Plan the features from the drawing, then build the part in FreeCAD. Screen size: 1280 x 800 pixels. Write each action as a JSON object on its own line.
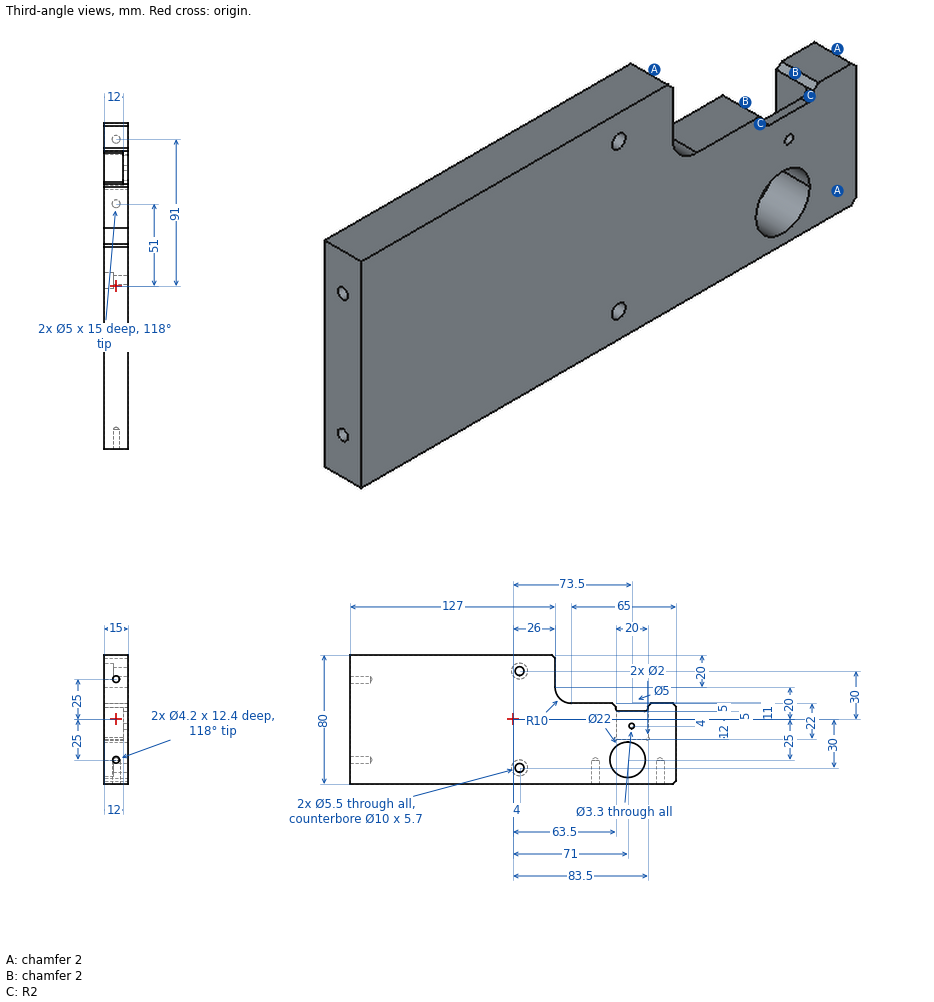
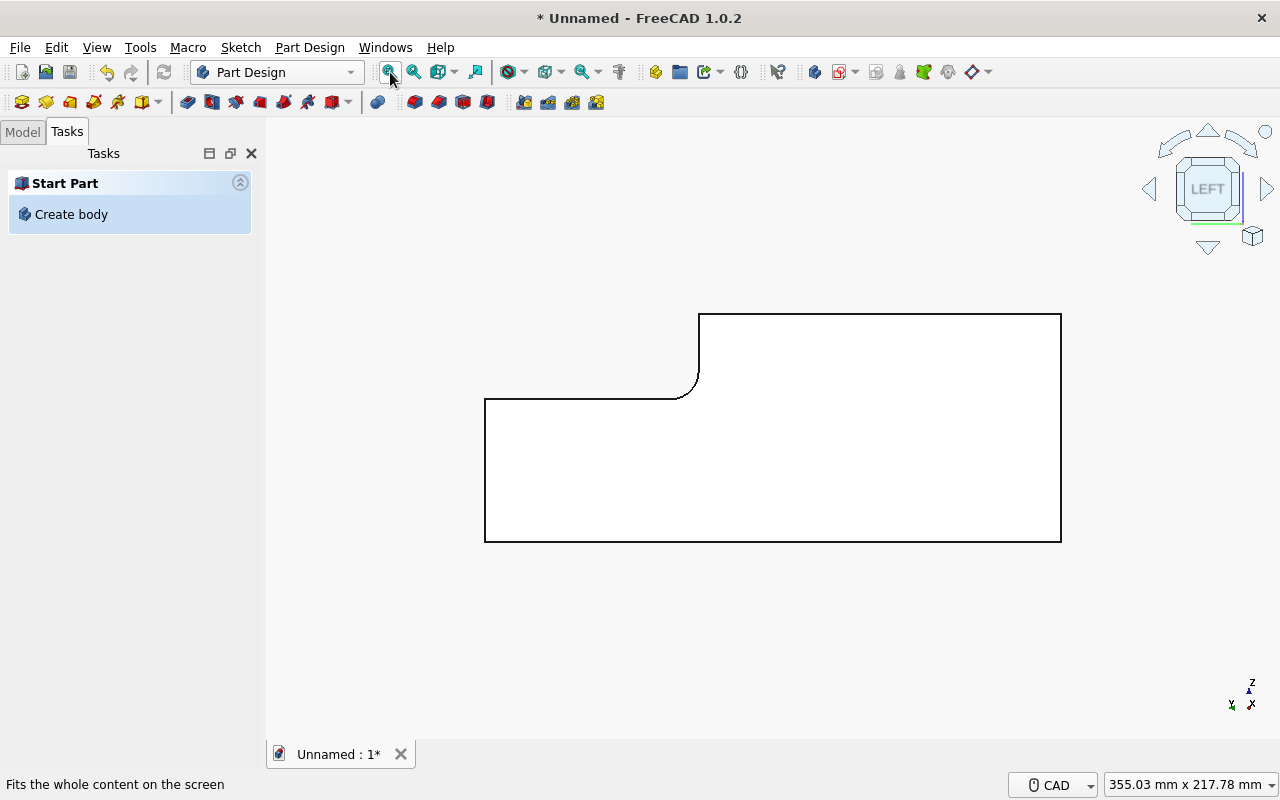
{"action": "left_click", "coordinate": [855, 427]}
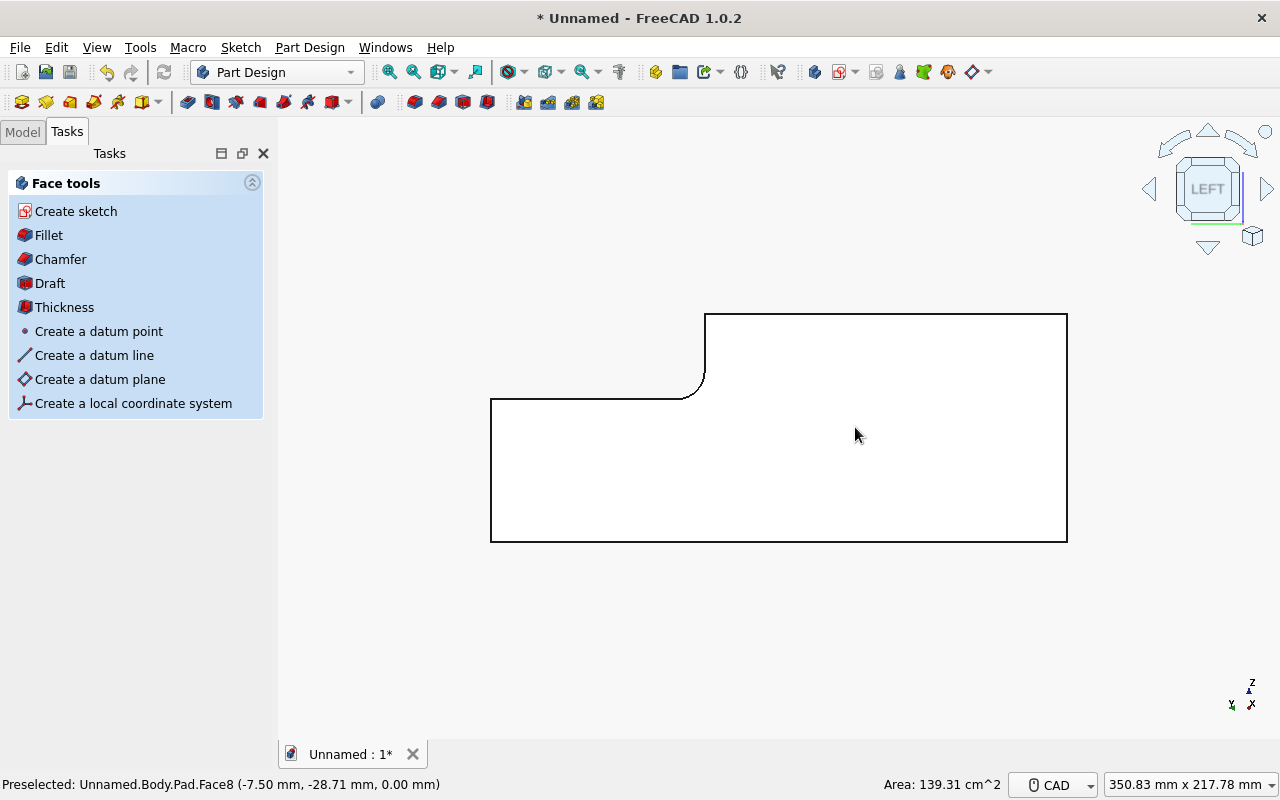
{"action": "left_click", "coordinate": [840, 72]}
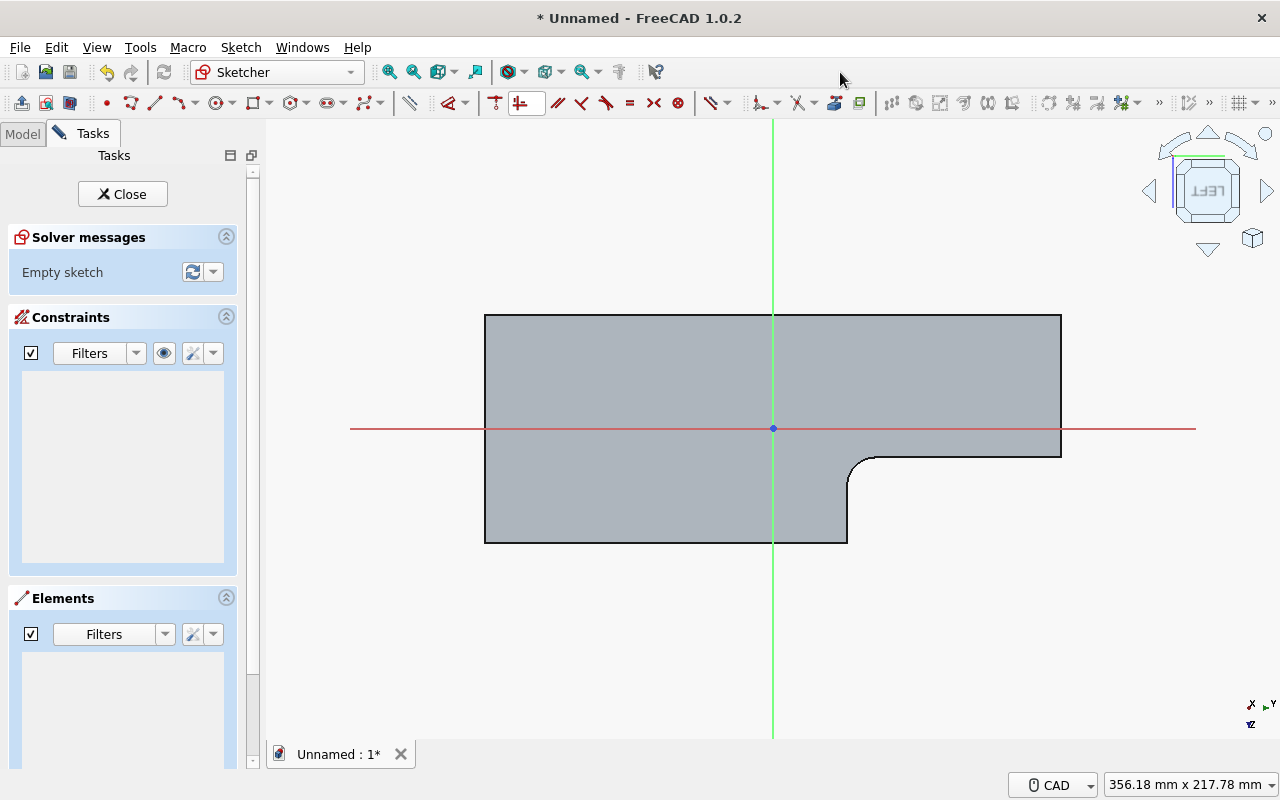
{"action": "scroll", "coordinate": [1029, 344], "scroll_direction": "up", "scroll_amount": 9}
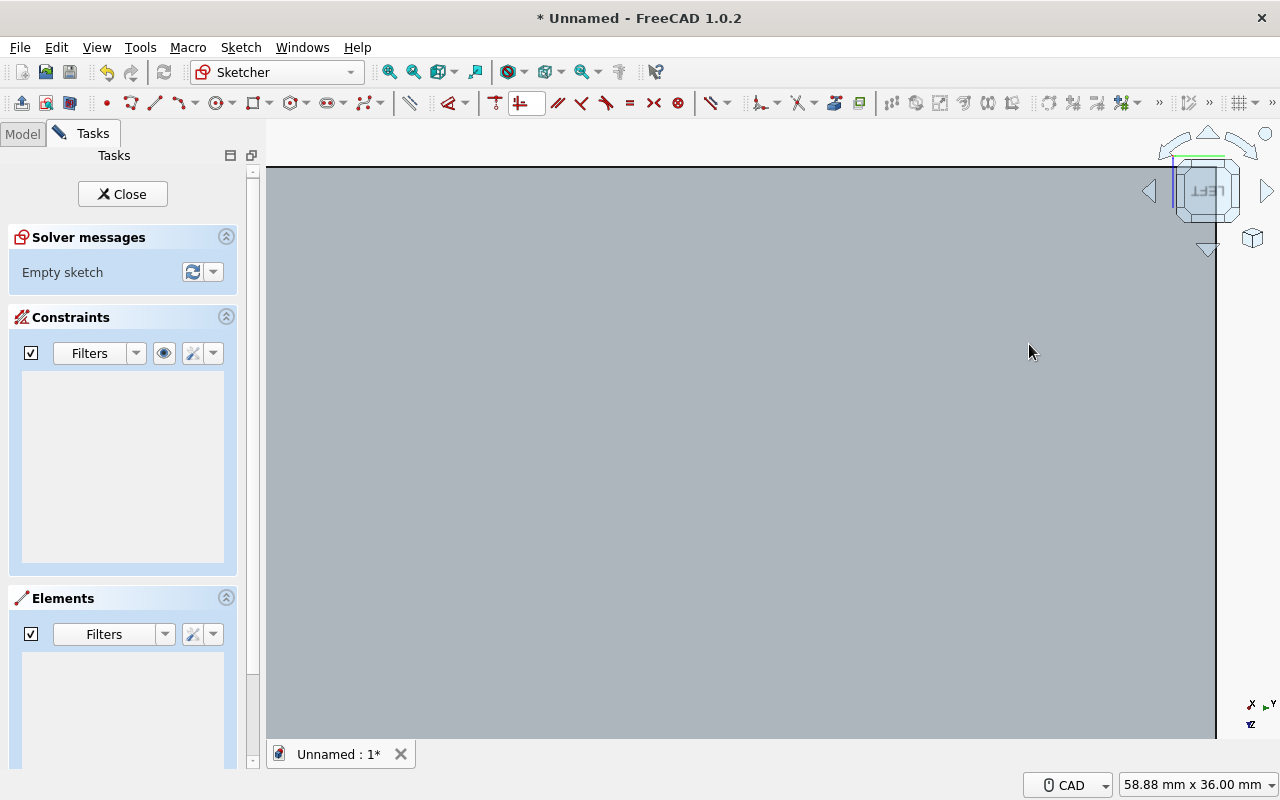
{"action": "left_click", "coordinate": [216, 104]}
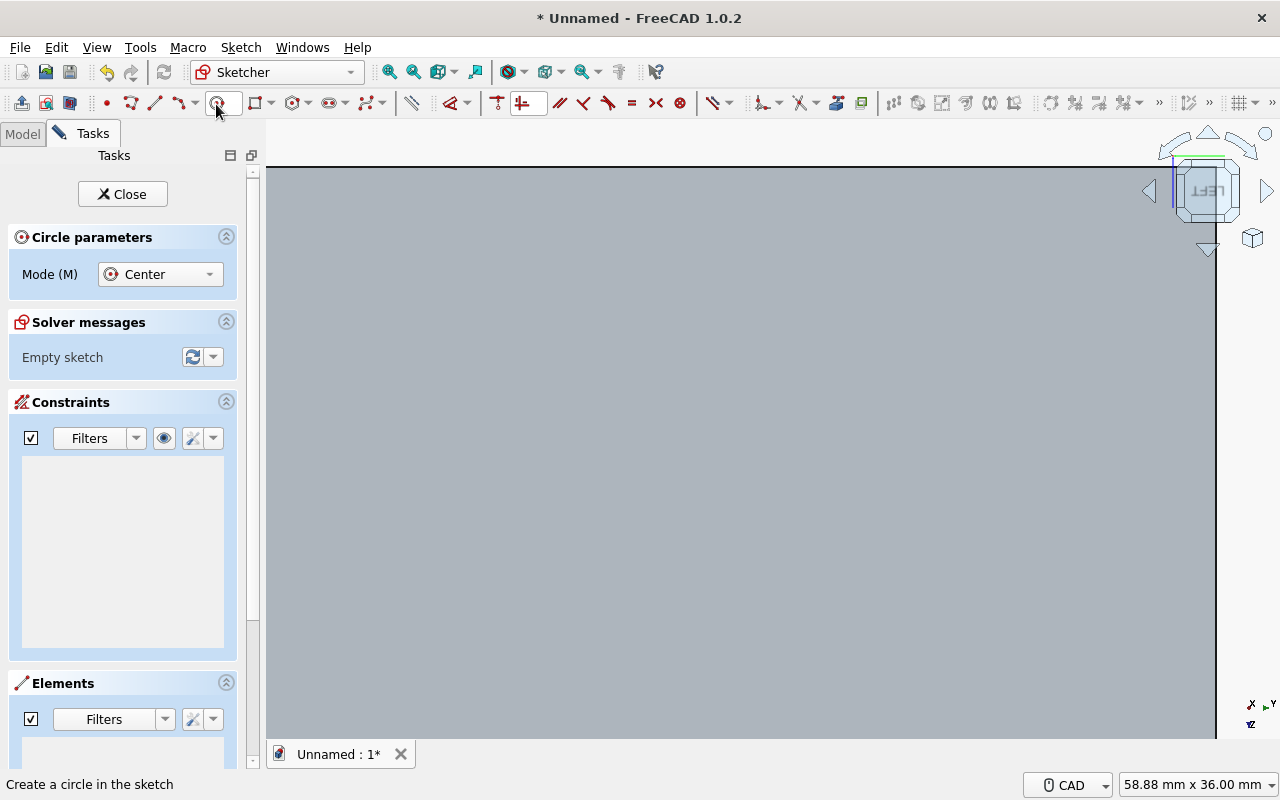
{"action": "left_click", "coordinate": [699, 426]}
{"action": "left_click", "coordinate": [833, 292]}
{"action": "key", "text": "Escape"}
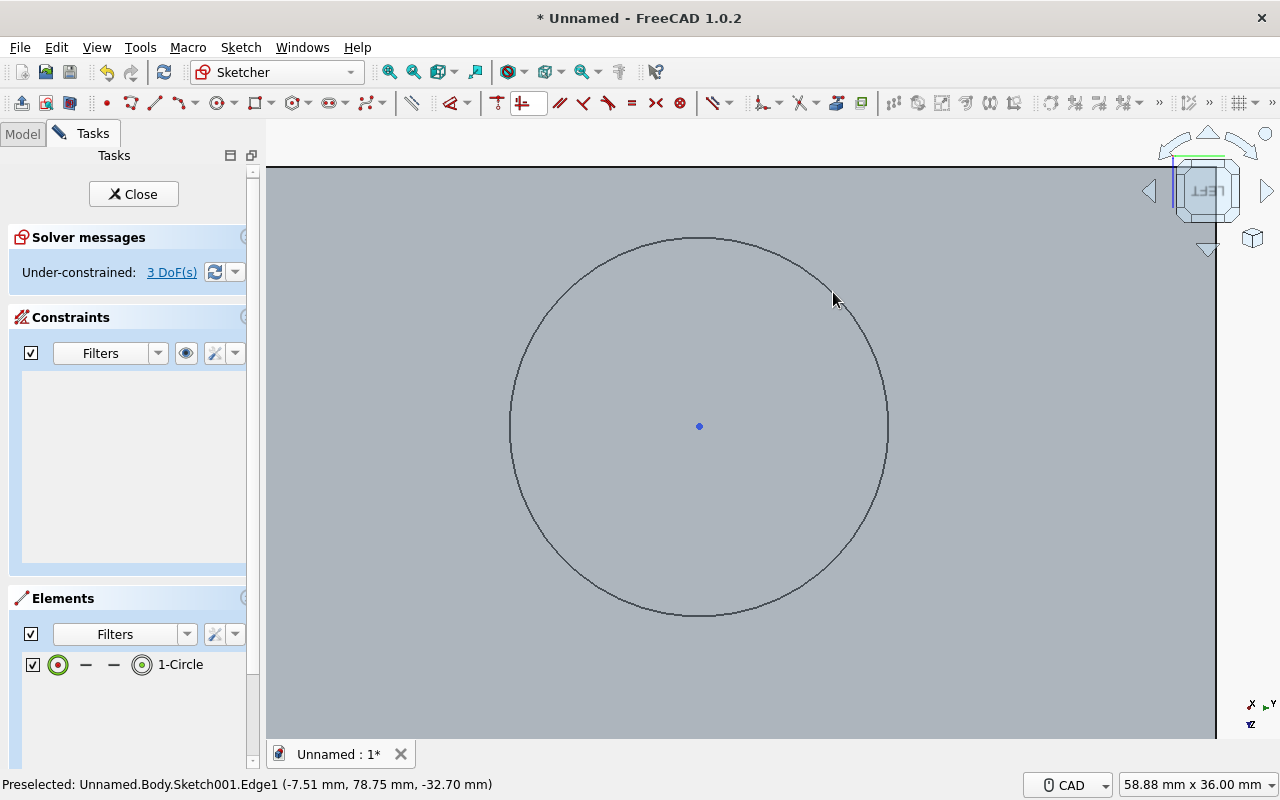
{"action": "left_click", "coordinate": [450, 104]}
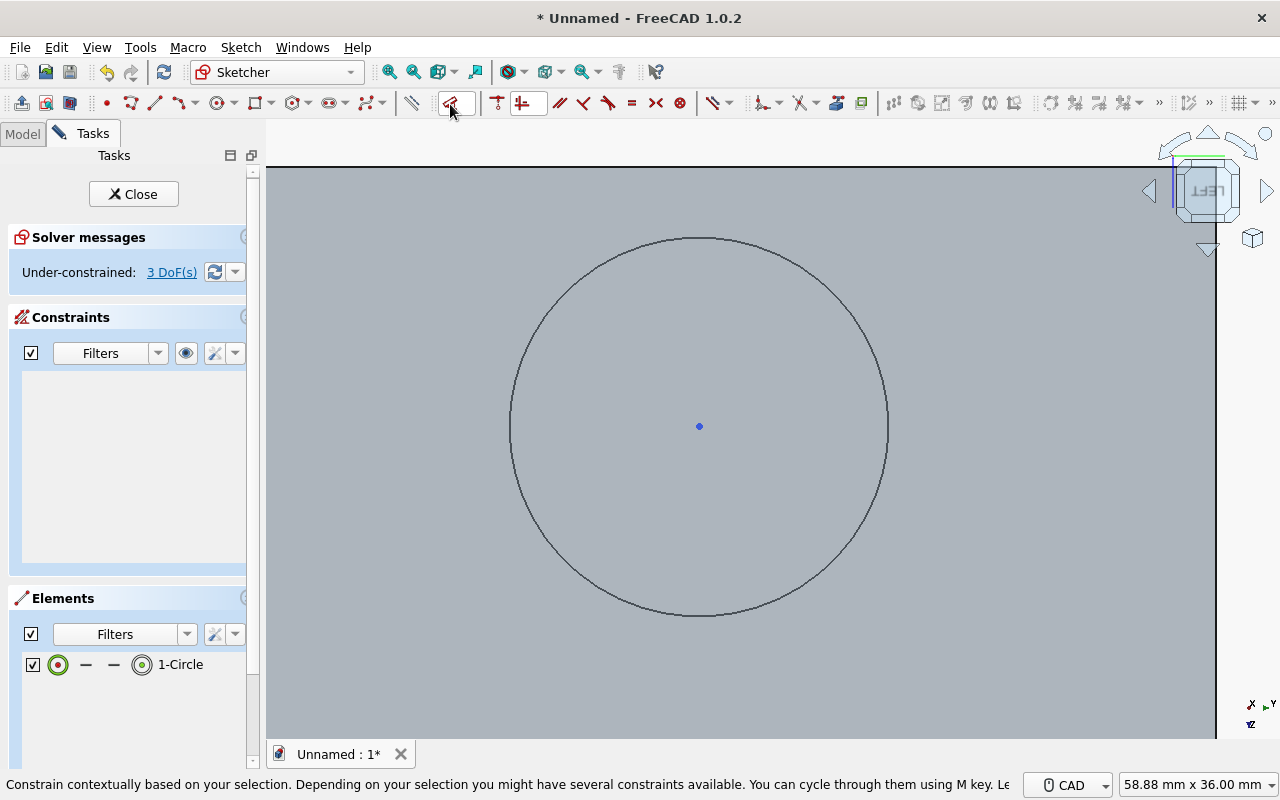
{"action": "left_click", "coordinate": [833, 293]}
{"action": "left_click", "coordinate": [856, 270]}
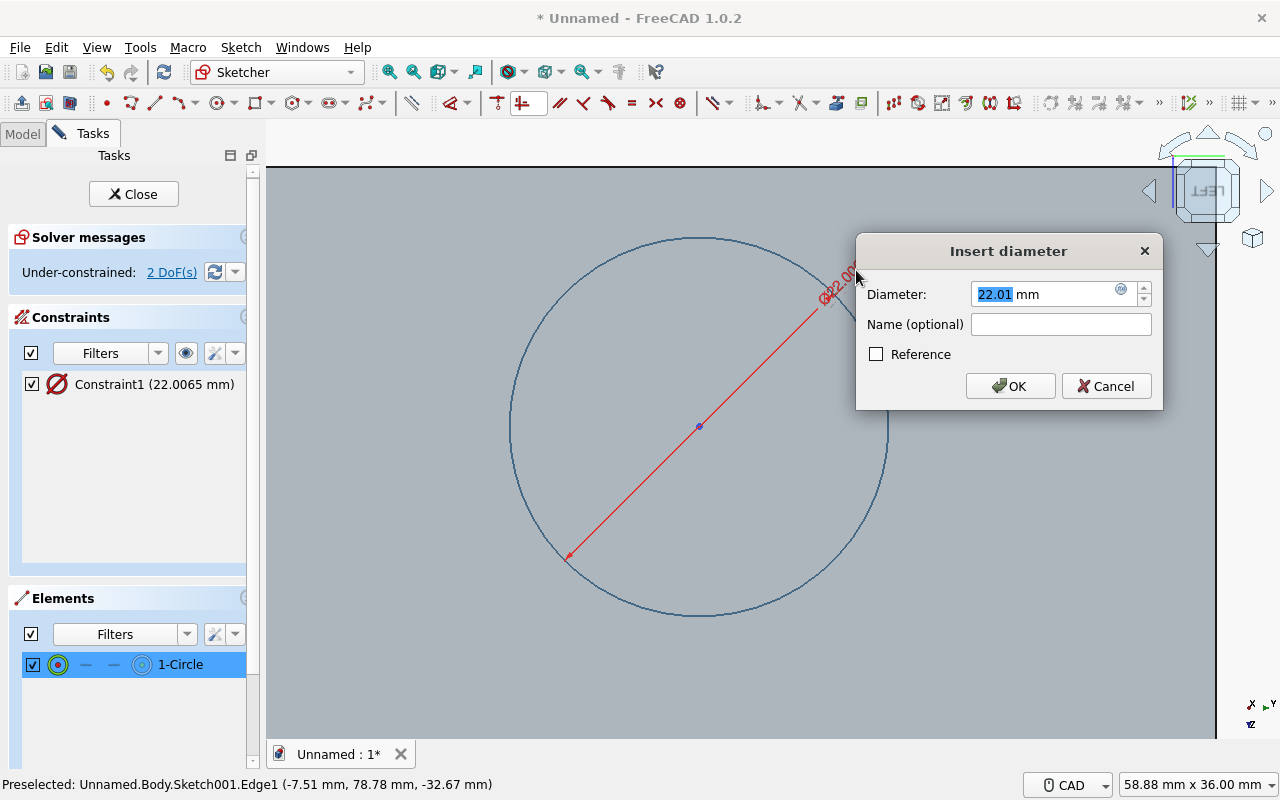
{"action": "type", "text": "22"}
{"action": "key", "text": "Return"}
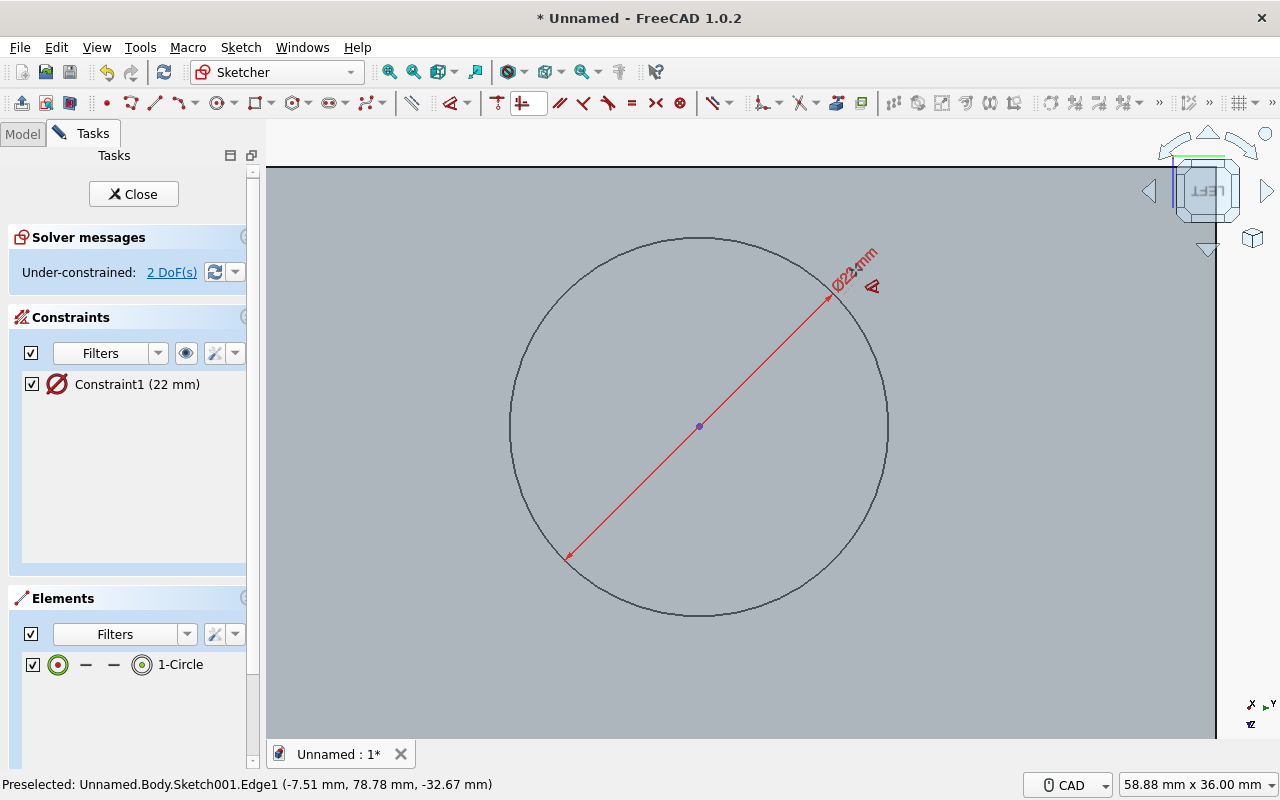
{"action": "left_click", "coordinate": [699, 427]}
{"action": "left_click", "coordinate": [497, 393]}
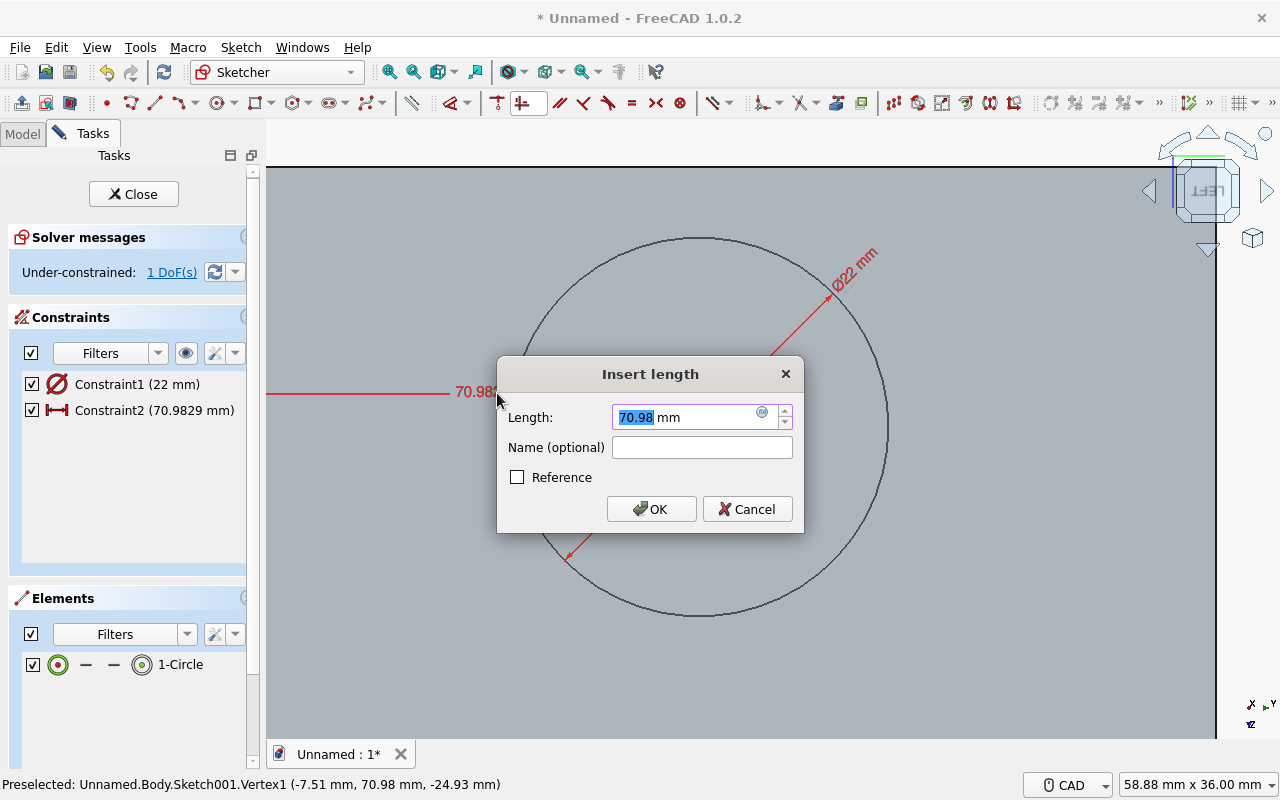
{"action": "type", "text": "71"}
{"action": "key", "text": "Return"}